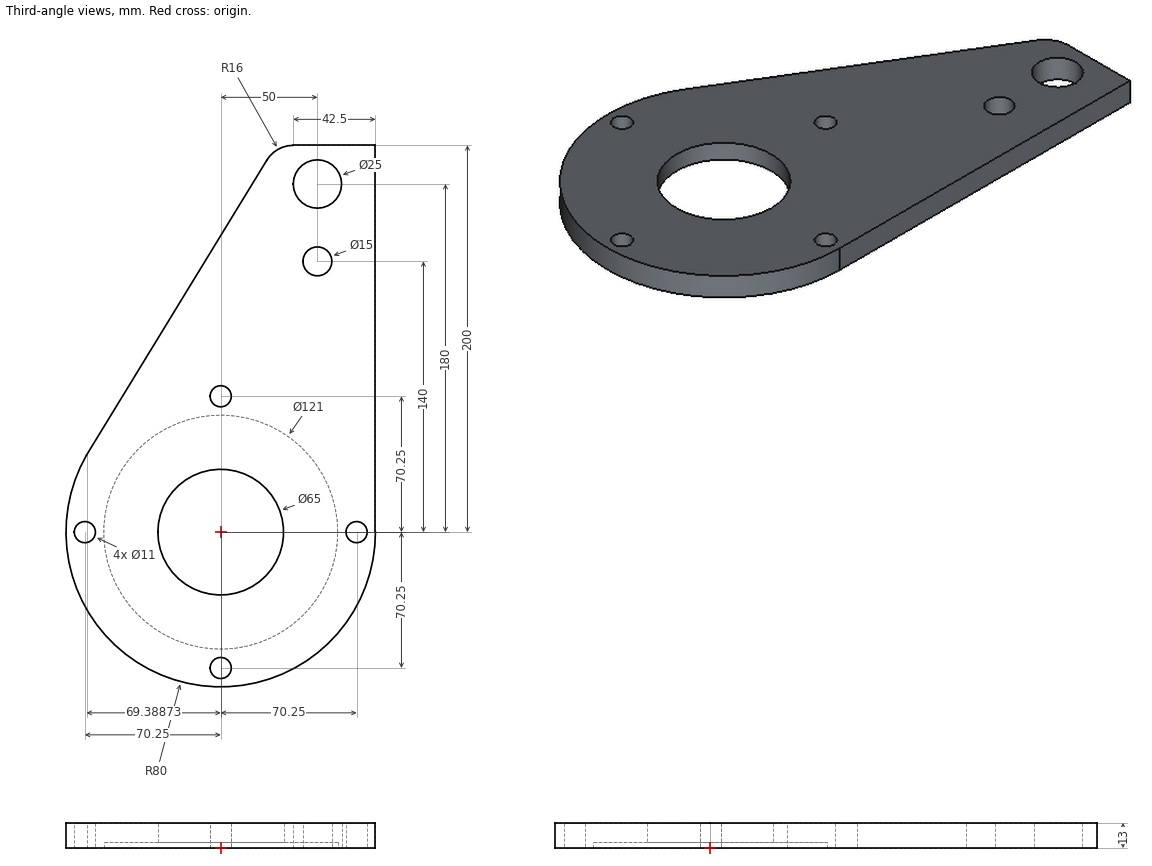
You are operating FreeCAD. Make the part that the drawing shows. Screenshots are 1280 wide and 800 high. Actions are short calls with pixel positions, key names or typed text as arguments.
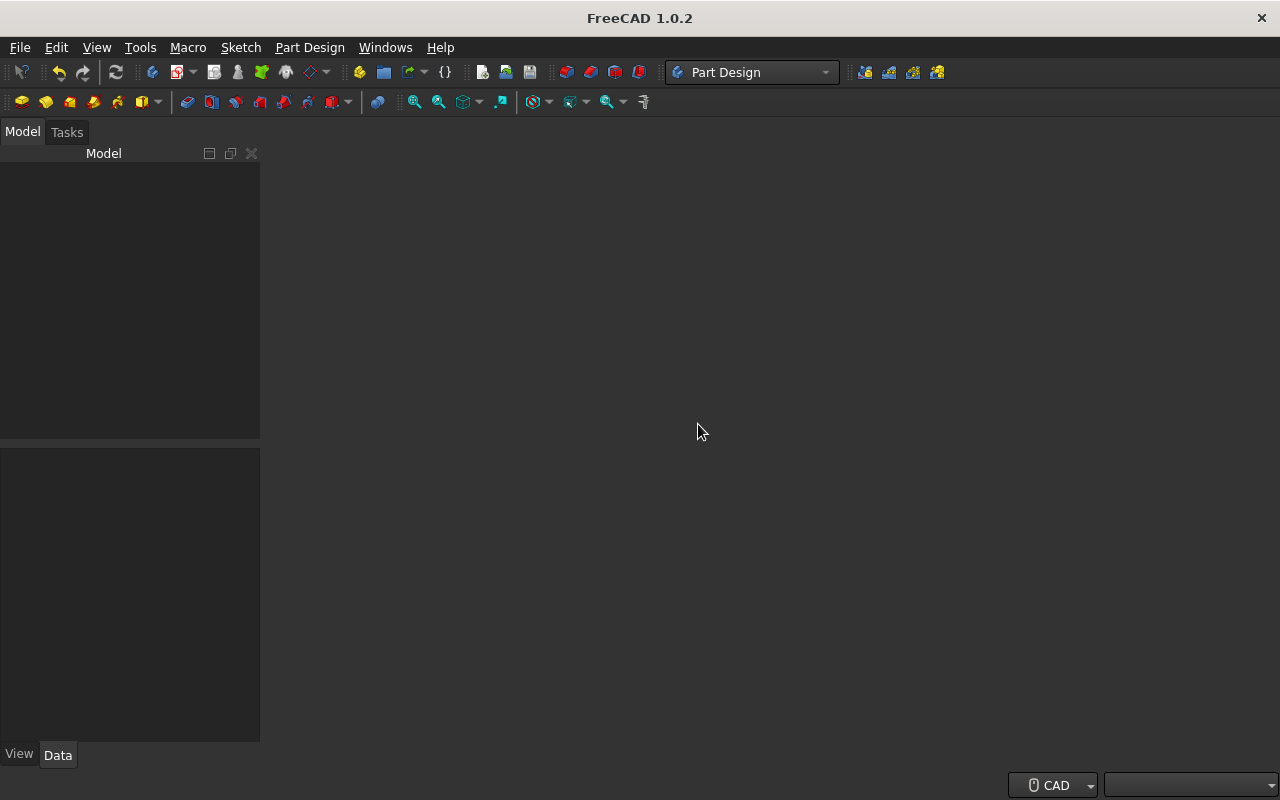
click(482, 72)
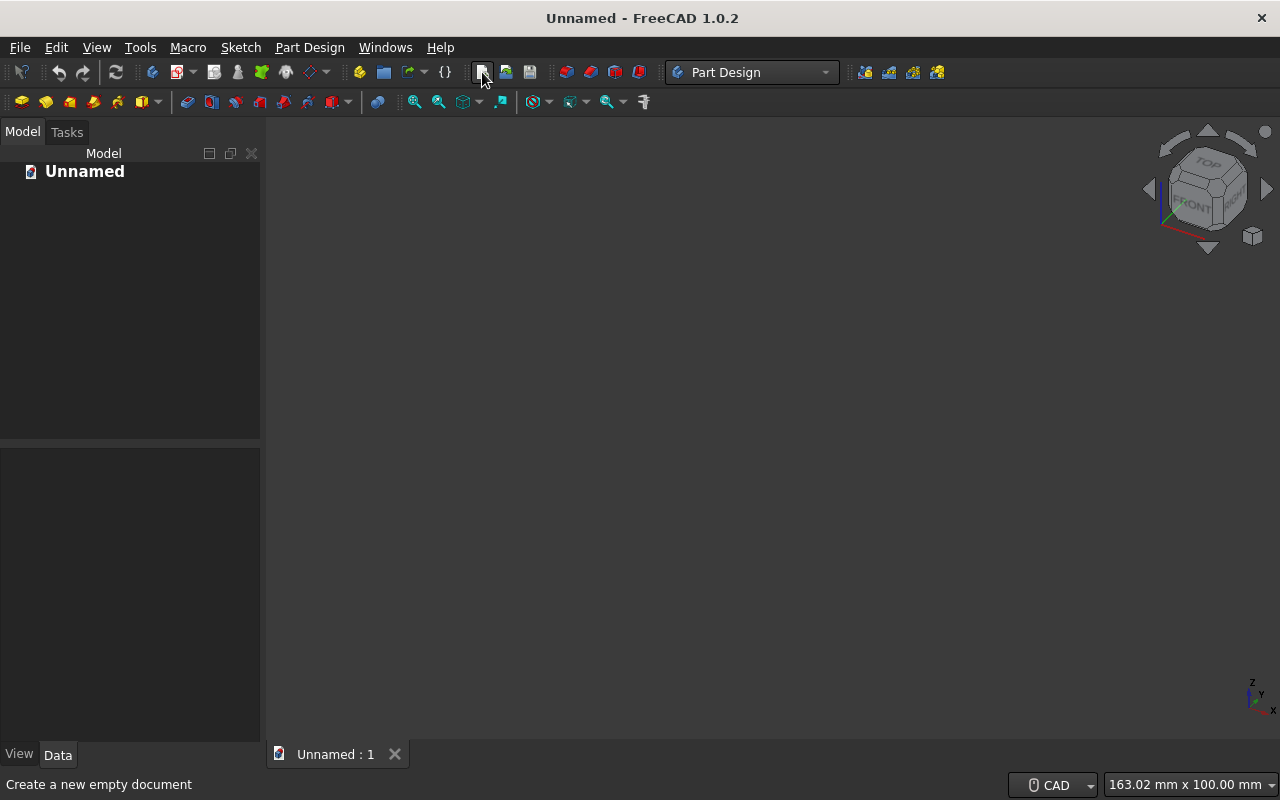
click(178, 72)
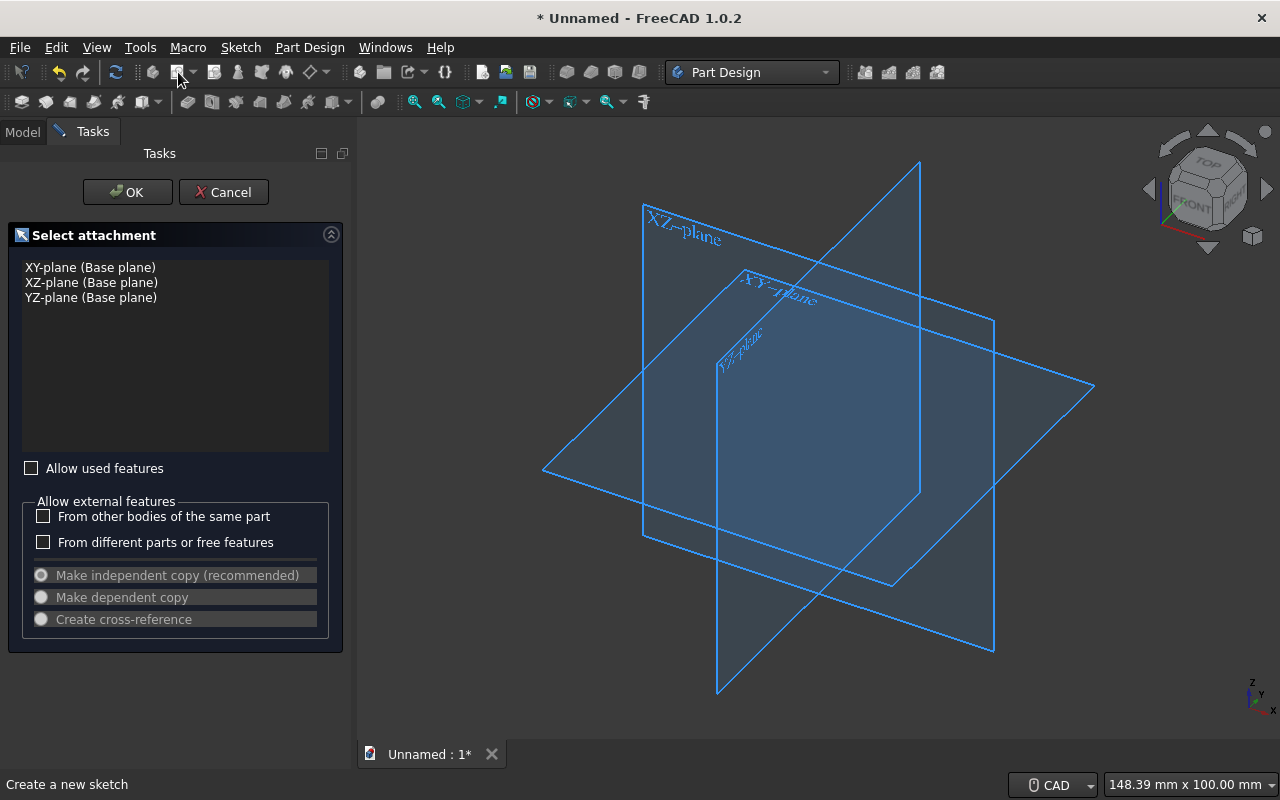
click(82, 268)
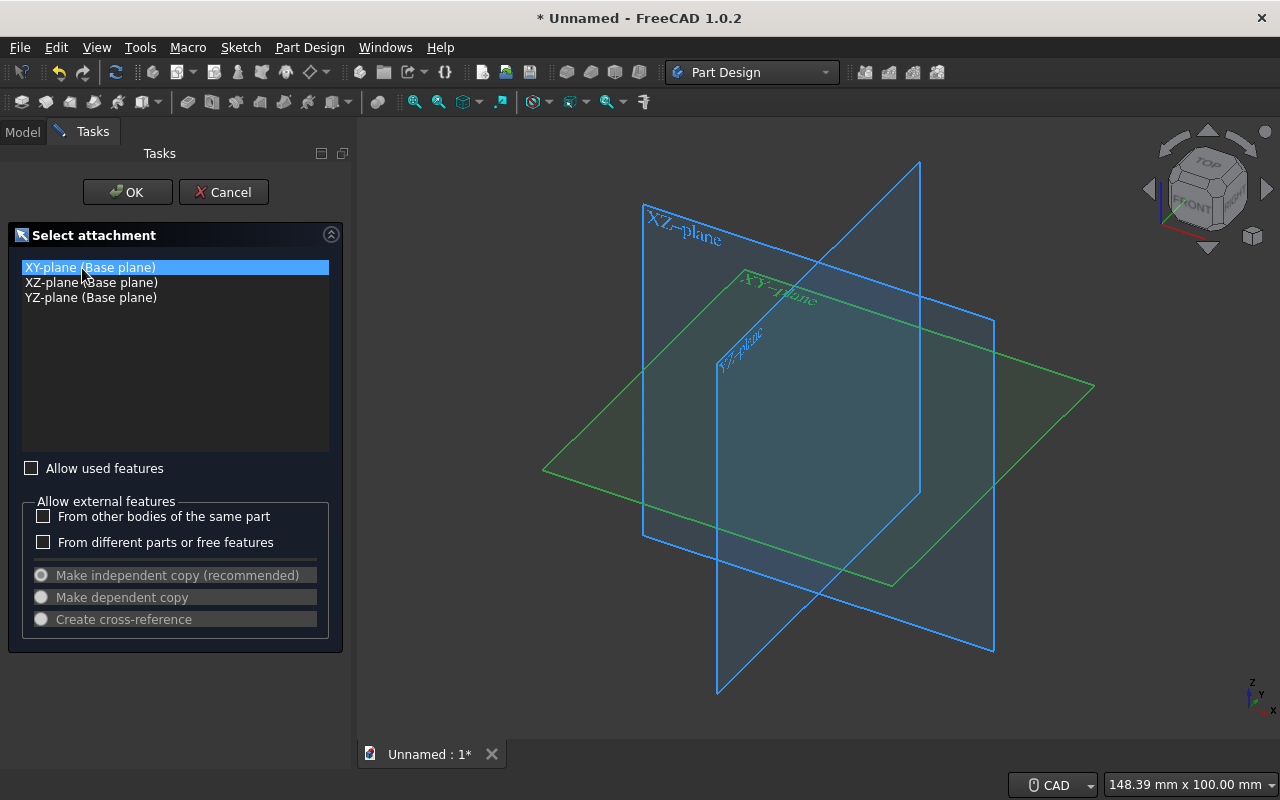
click(128, 192)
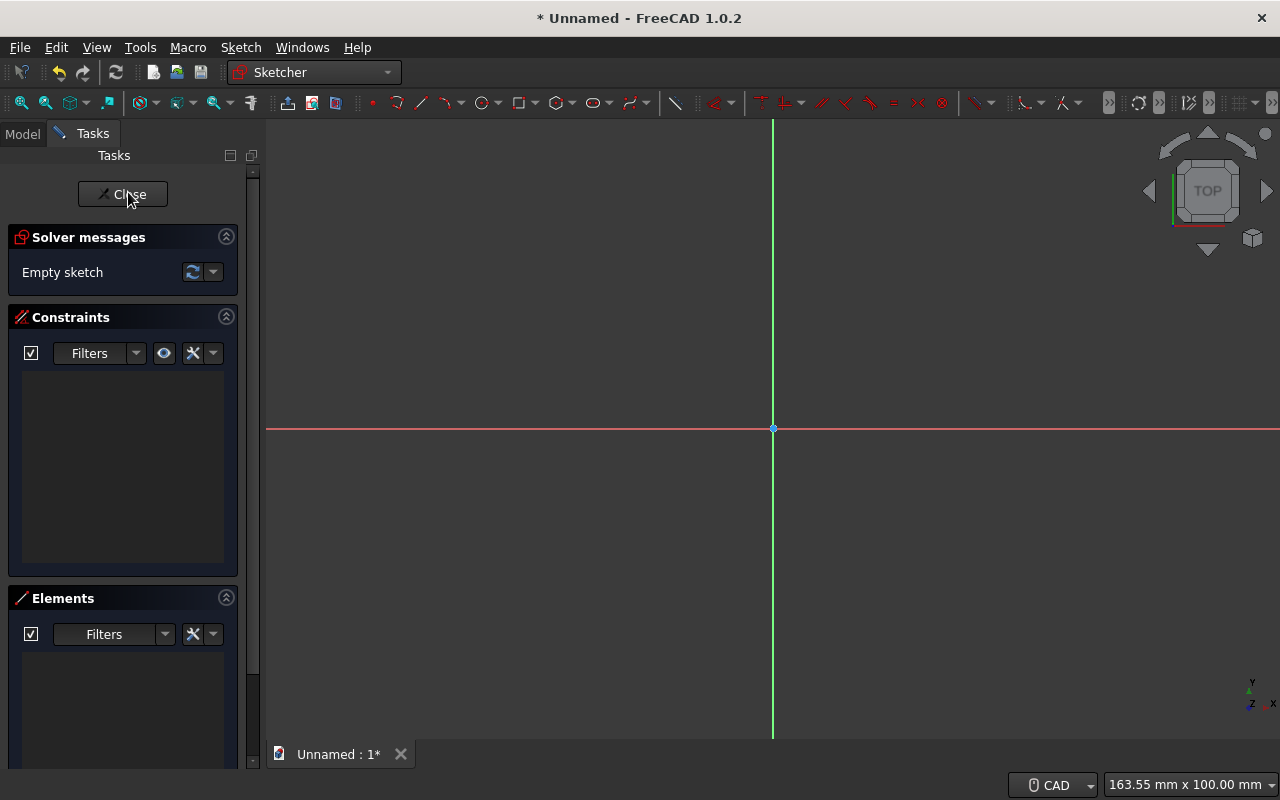
scroll(671, 553, down, 7)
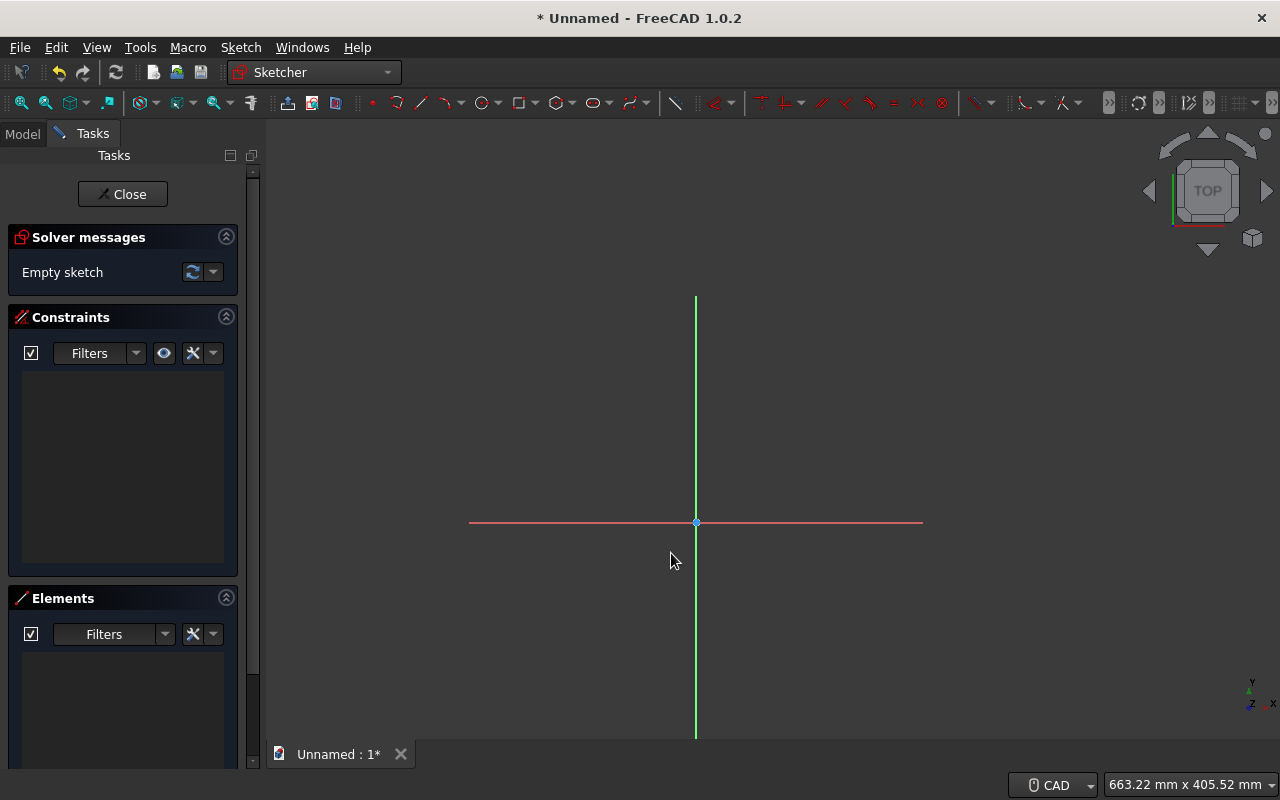
click(422, 104)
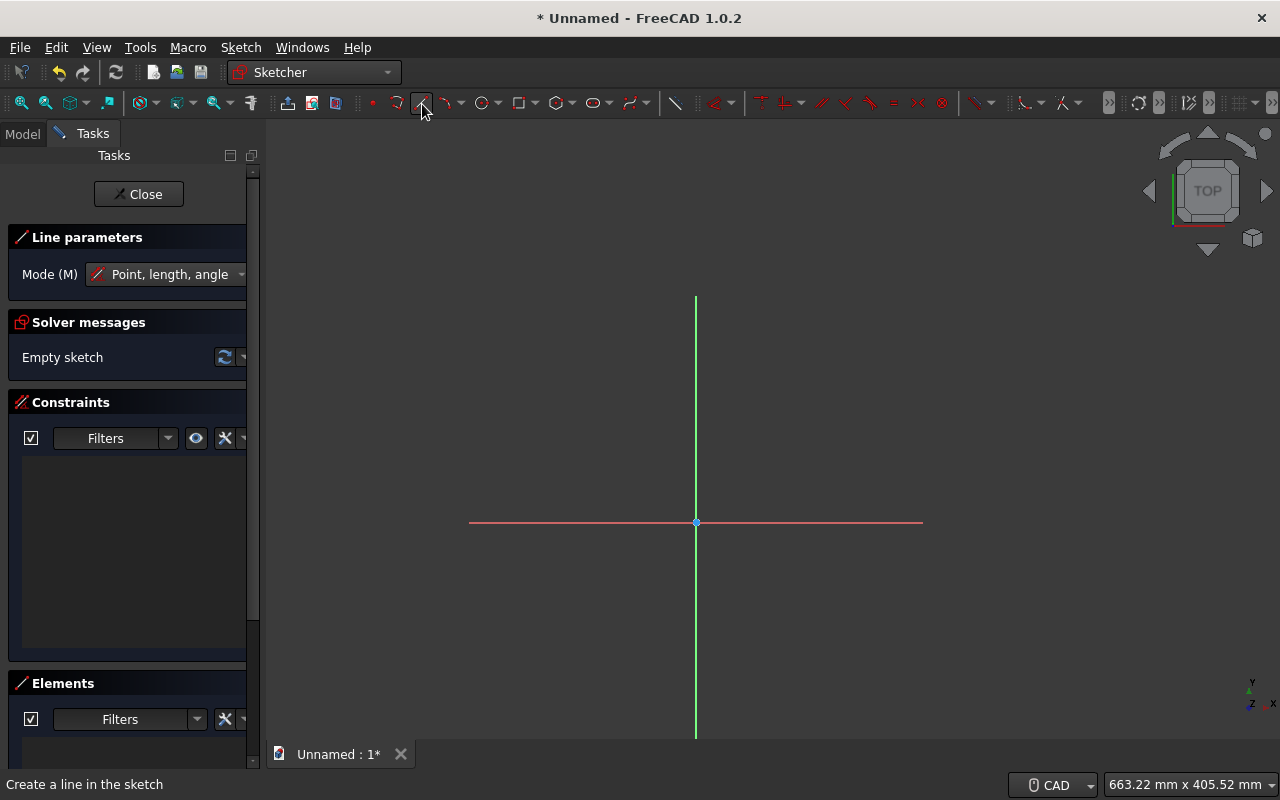
click(733, 229)
click(590, 462)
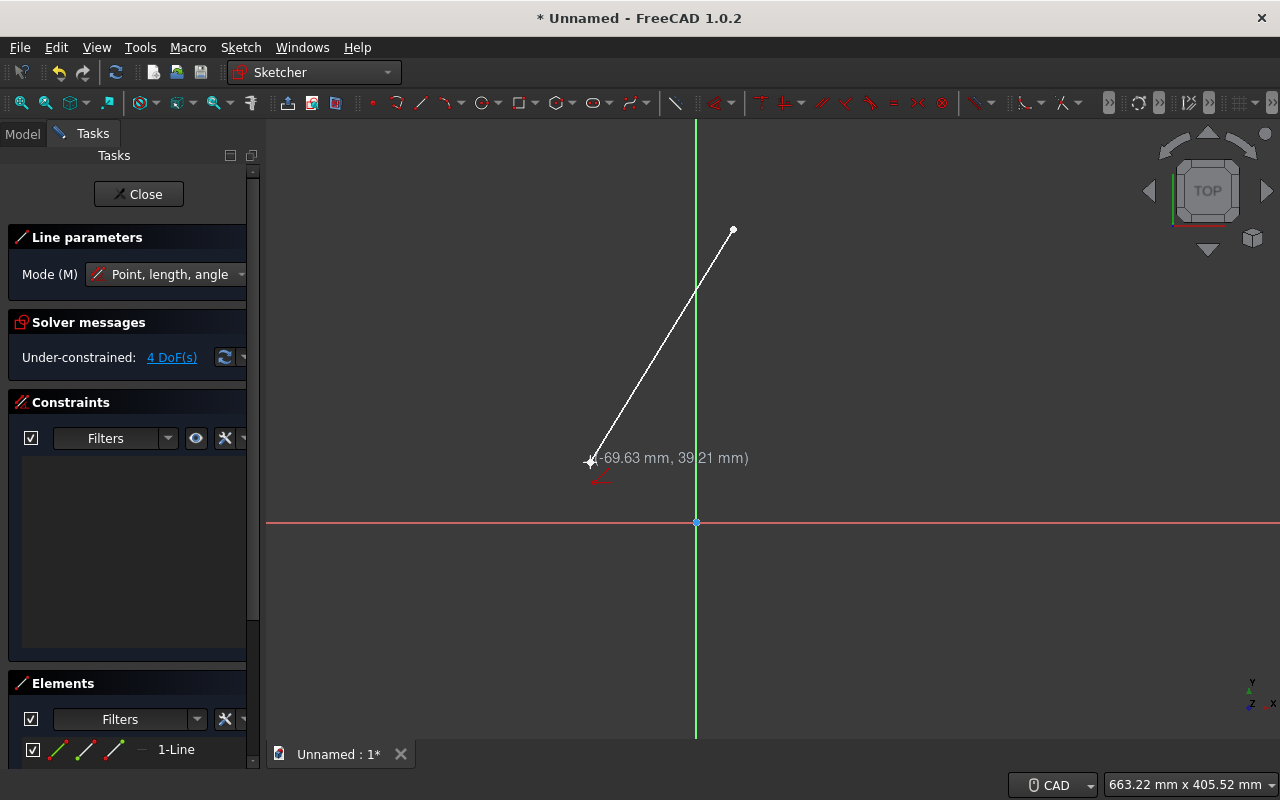
click(398, 104)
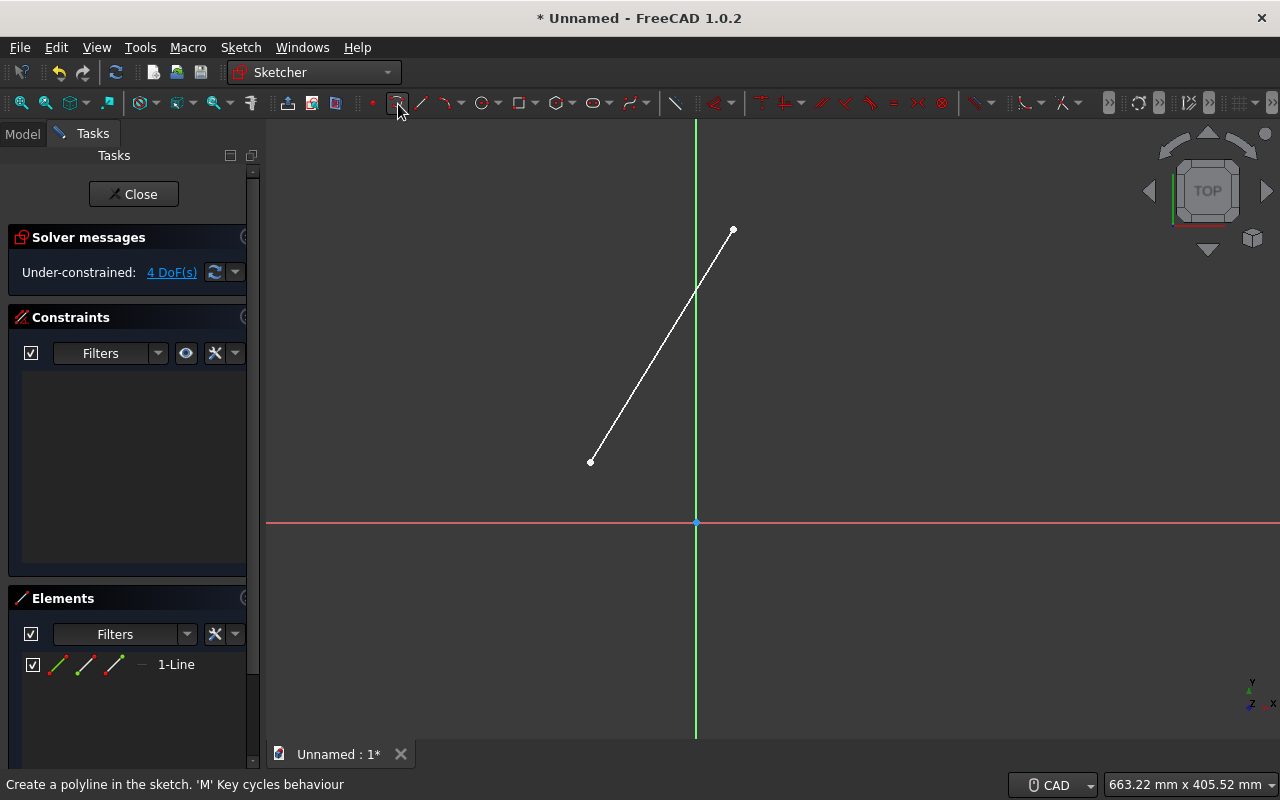
click(819, 523)
click(819, 217)
click(754, 217)
right_click(754, 217)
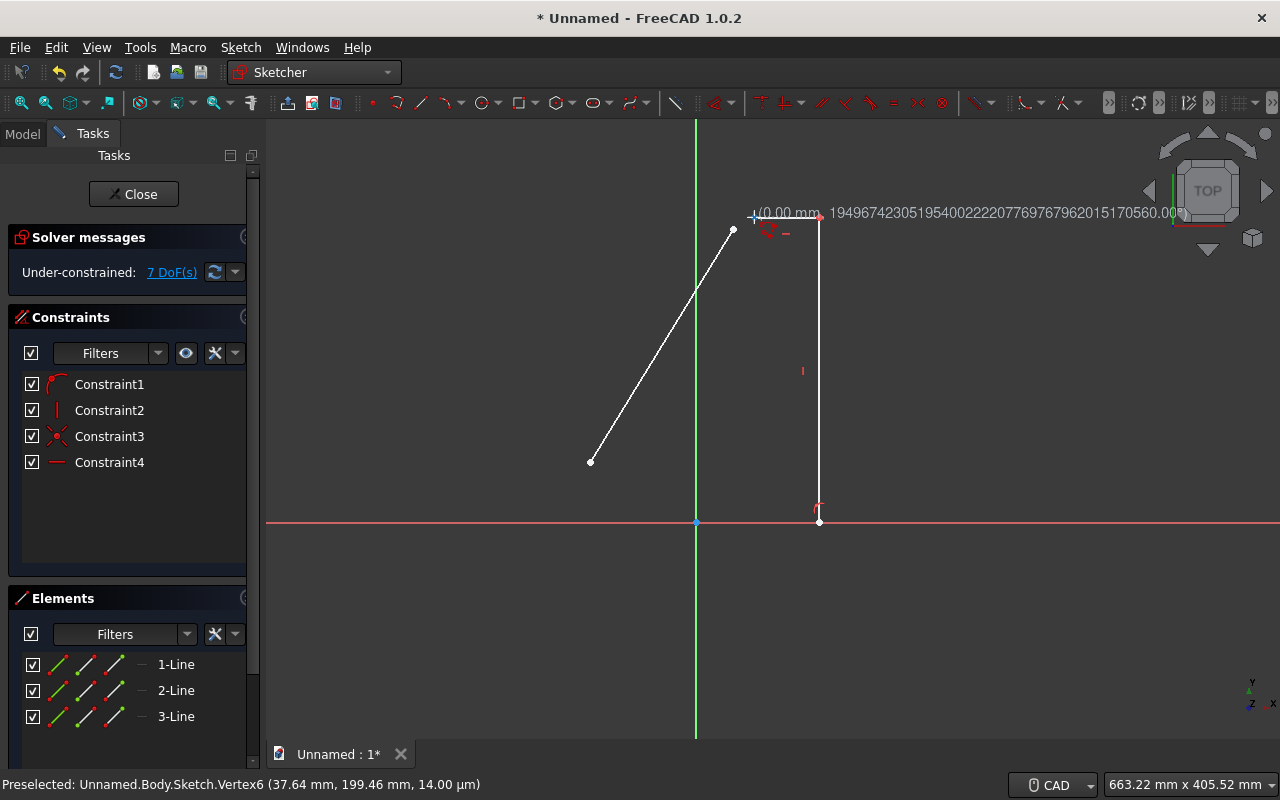
click(446, 104)